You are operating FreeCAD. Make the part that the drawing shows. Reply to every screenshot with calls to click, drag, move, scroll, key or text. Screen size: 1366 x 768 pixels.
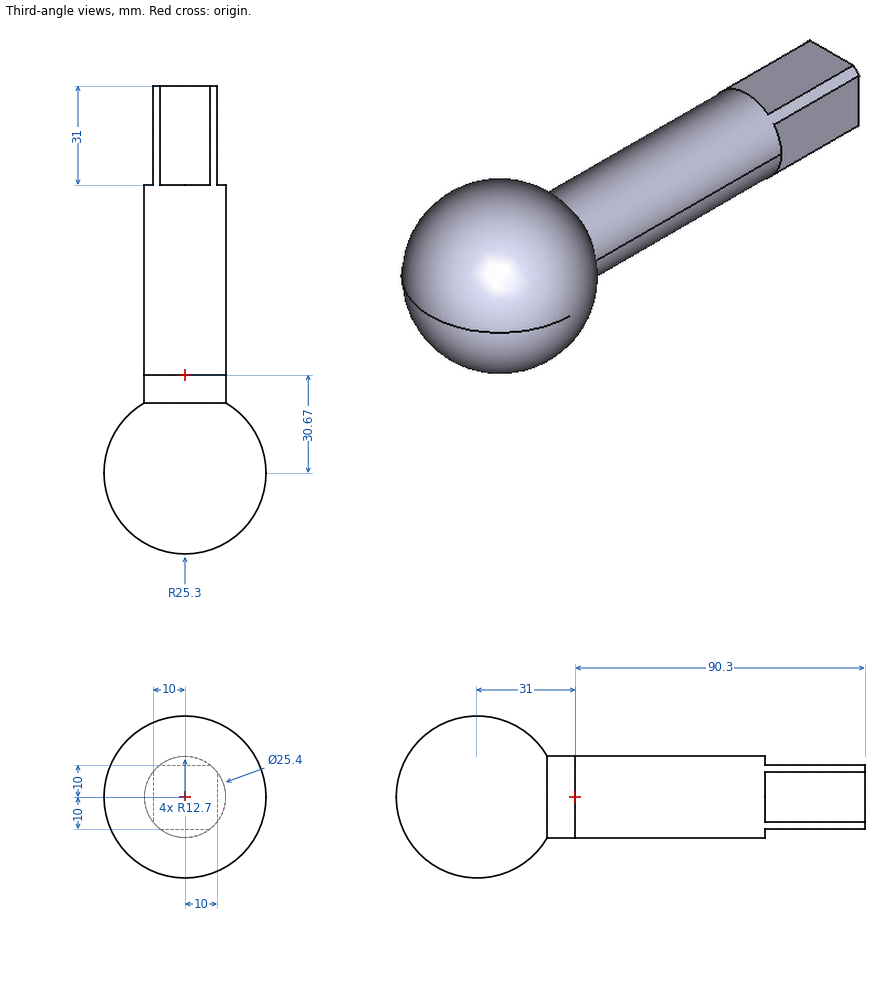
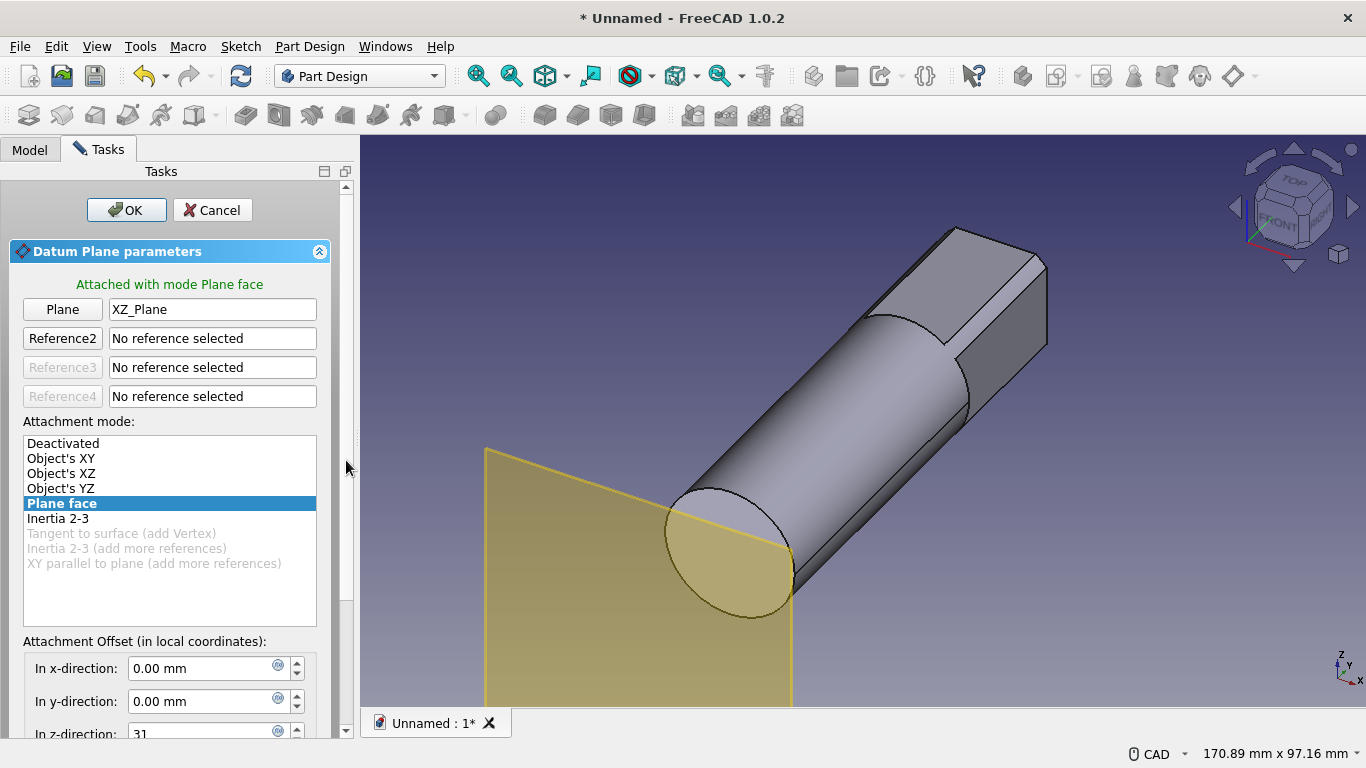
click(127, 210)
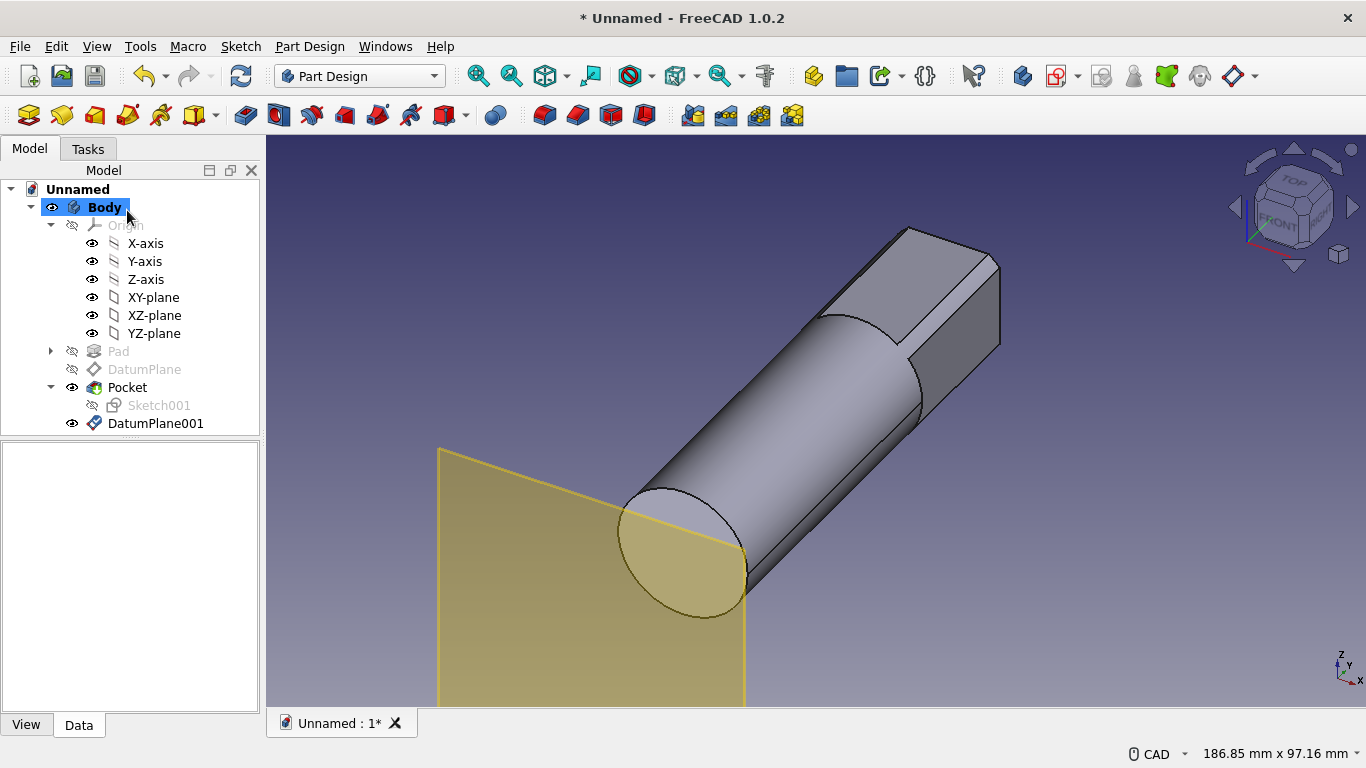
click(117, 423)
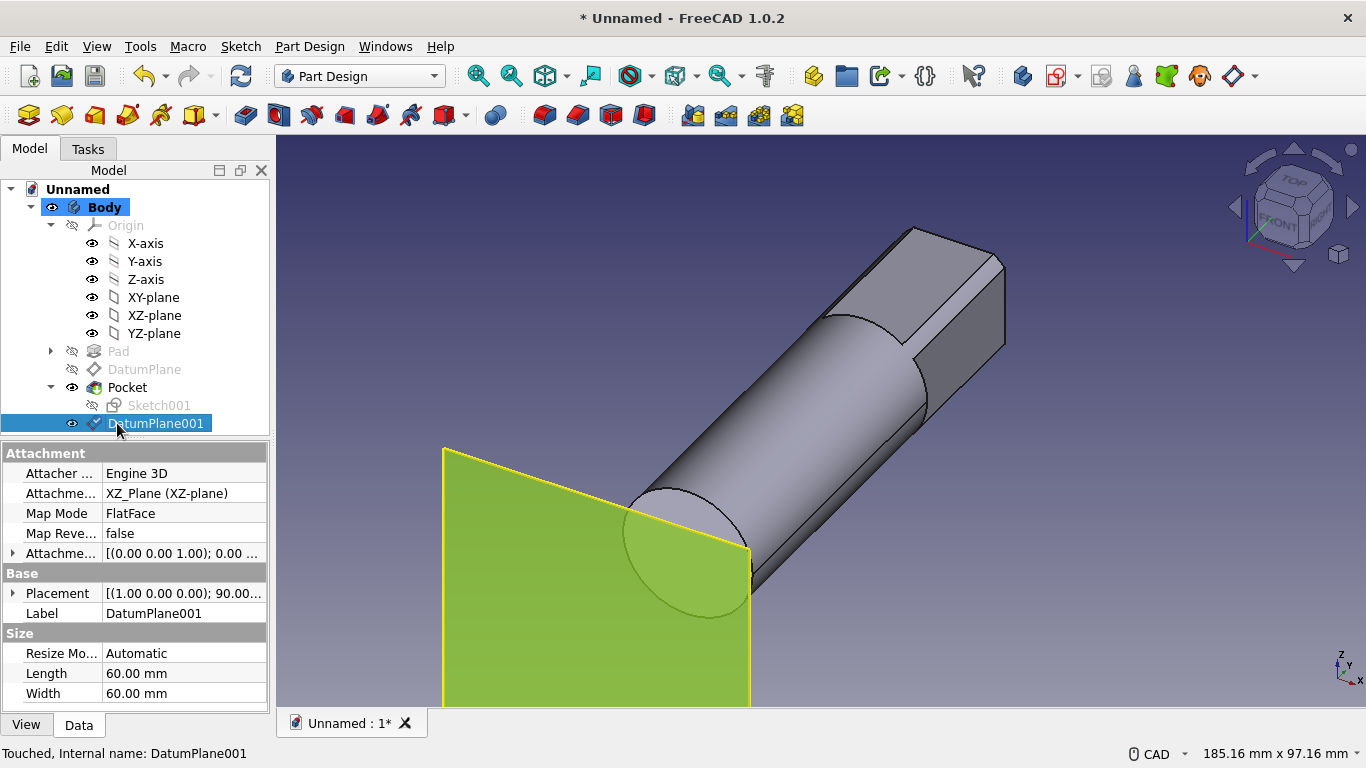
click(1056, 76)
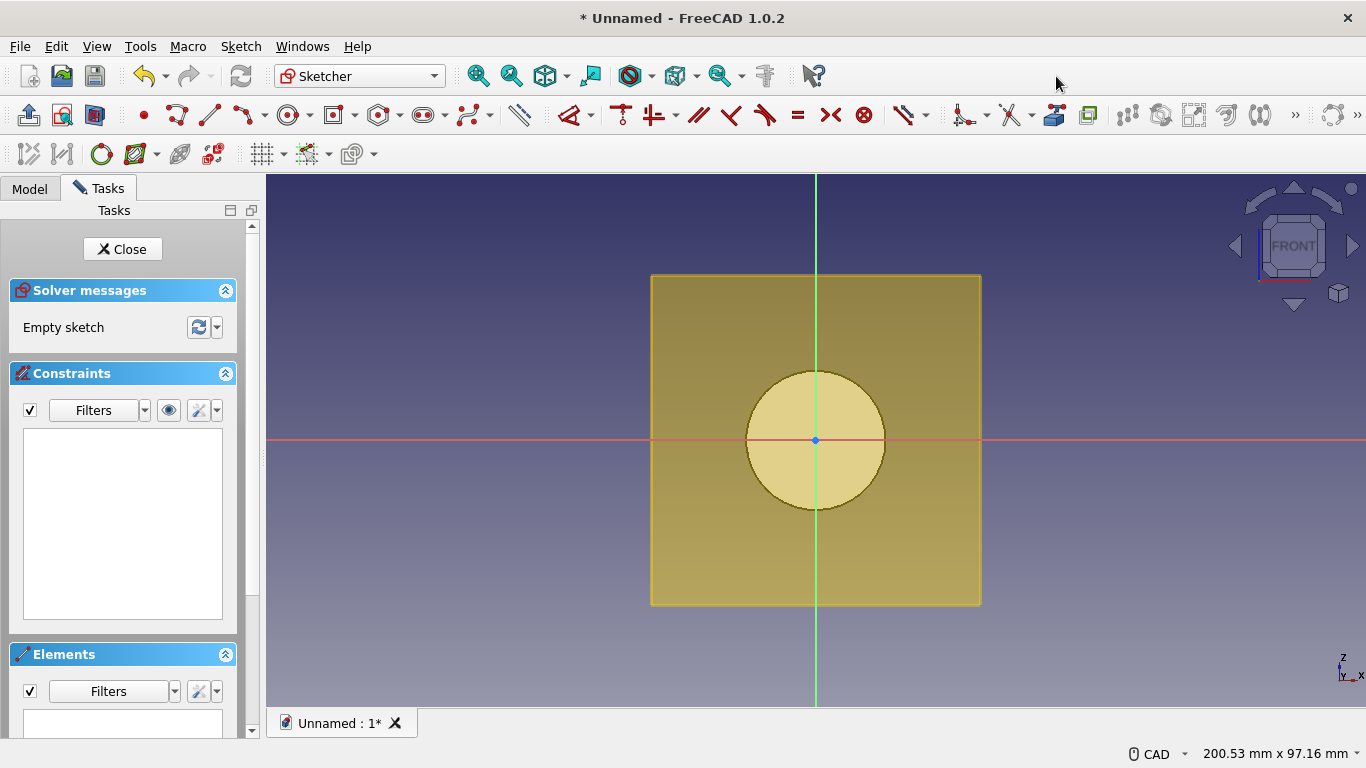
scroll(872, 440, up, 4)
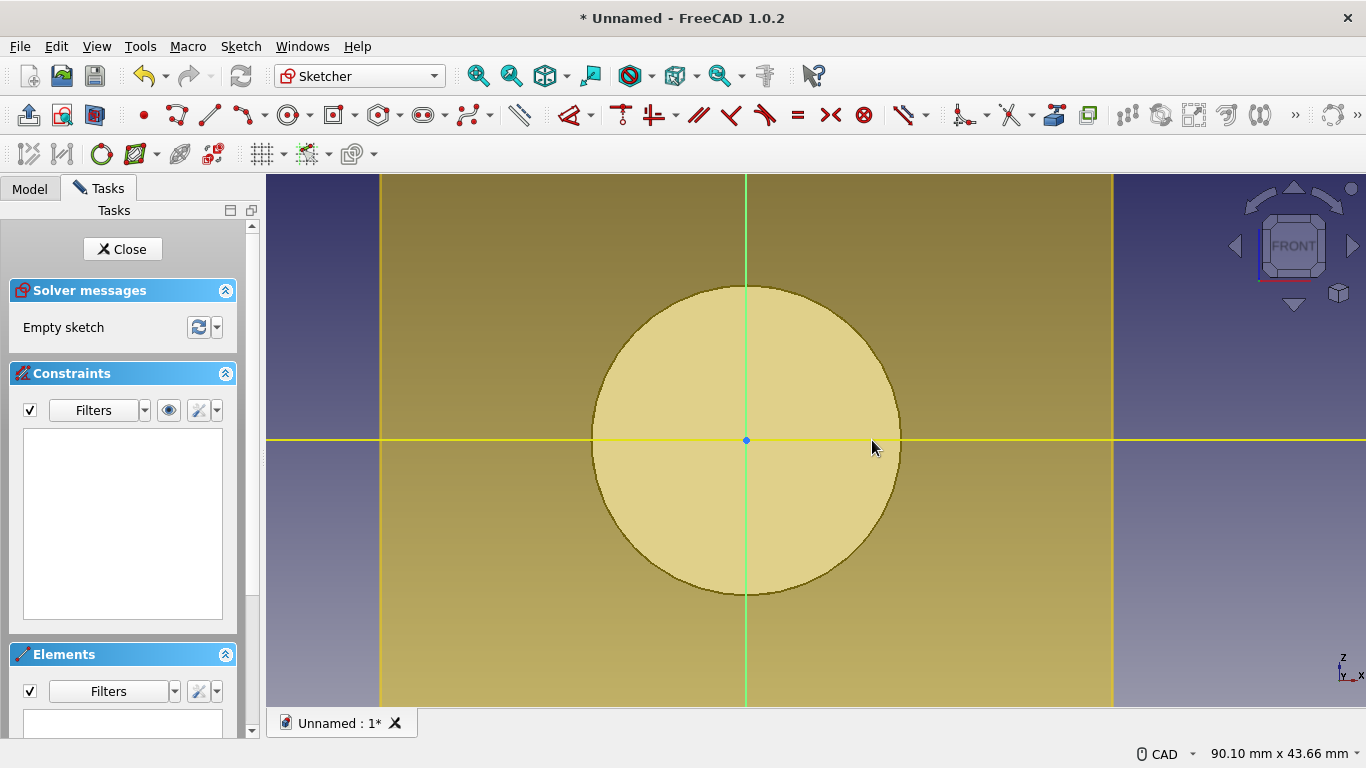
click(288, 116)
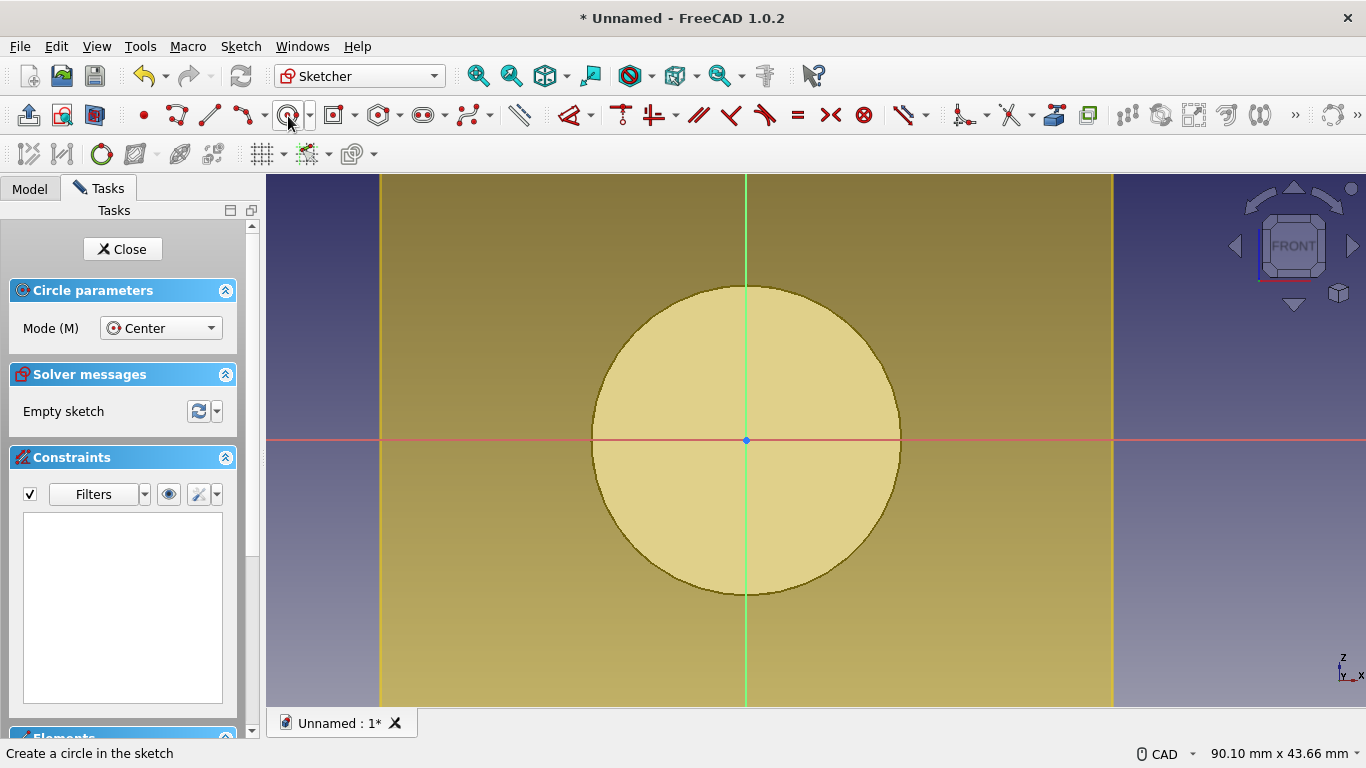
click(746, 440)
move(856, 331)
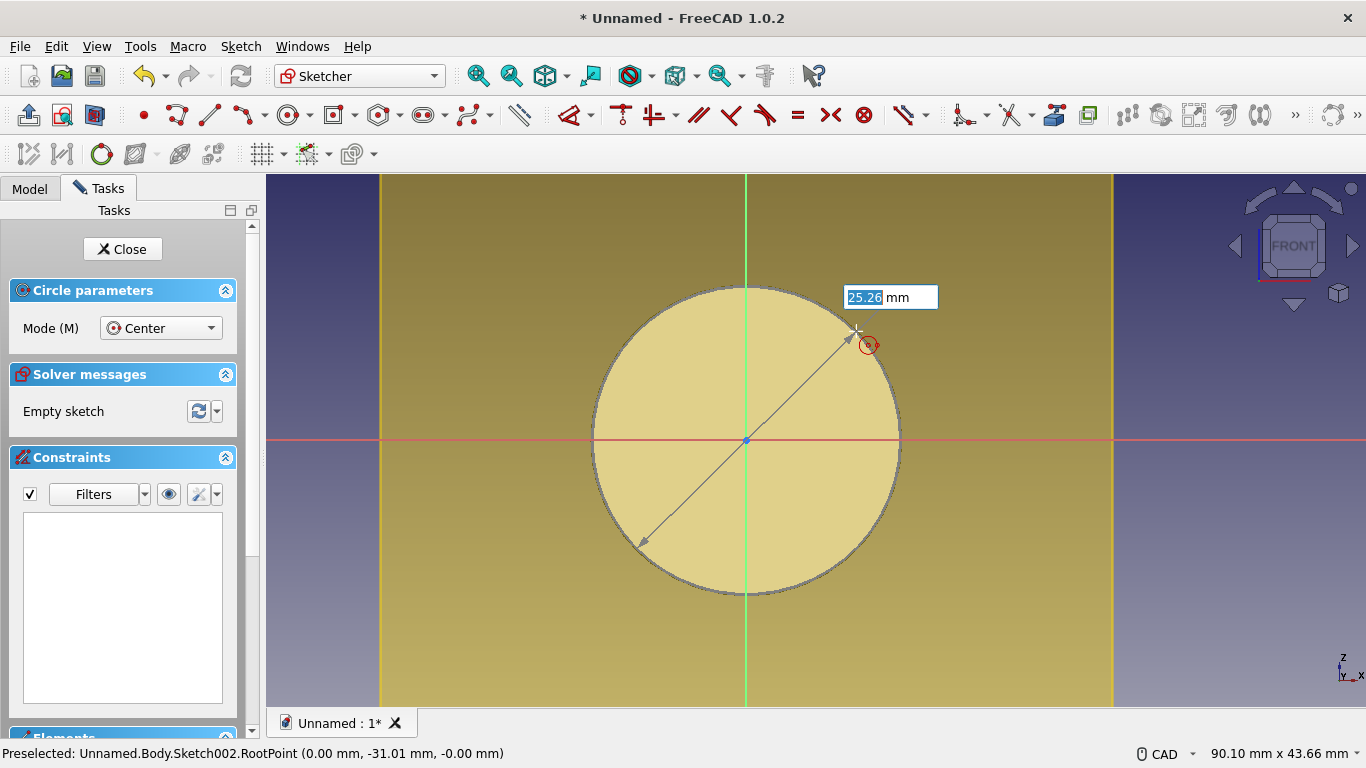
text(25.4)
key(Return)
key(Escape)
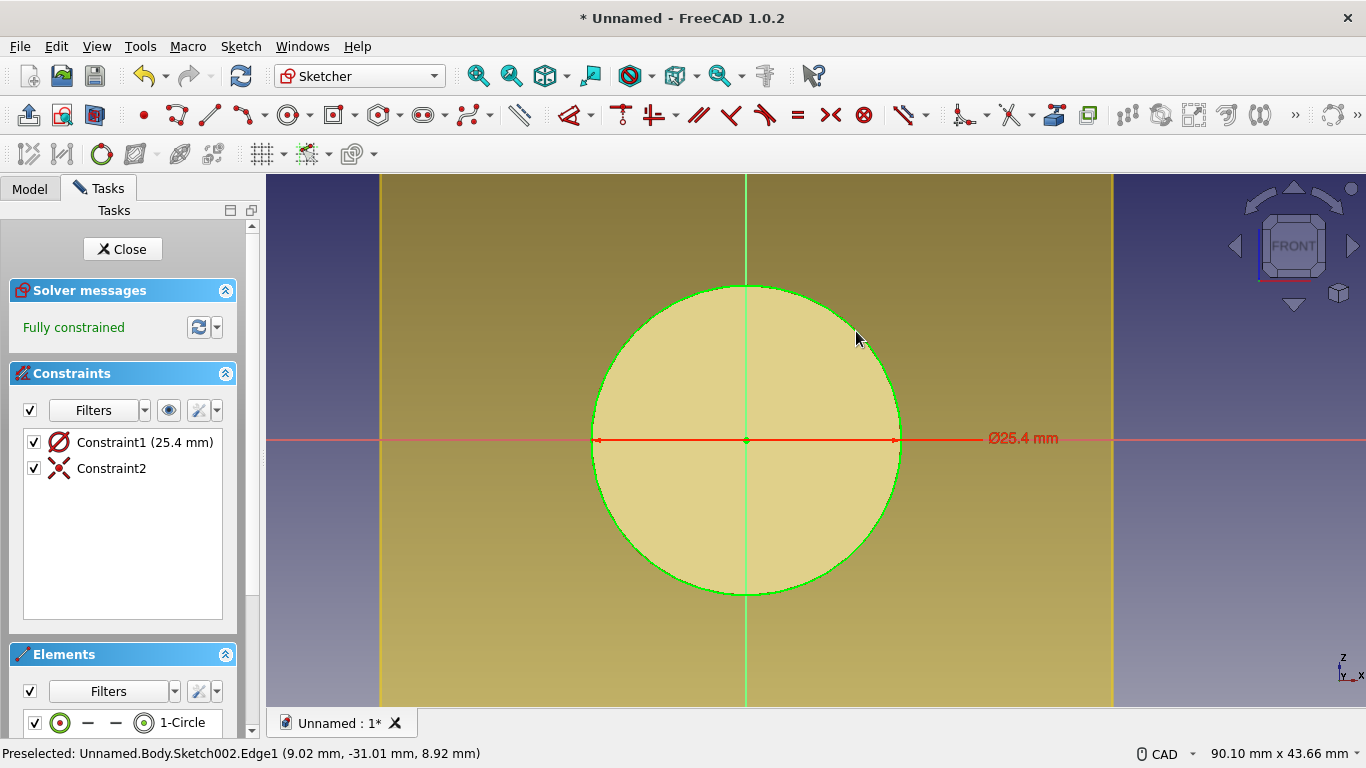
click(123, 249)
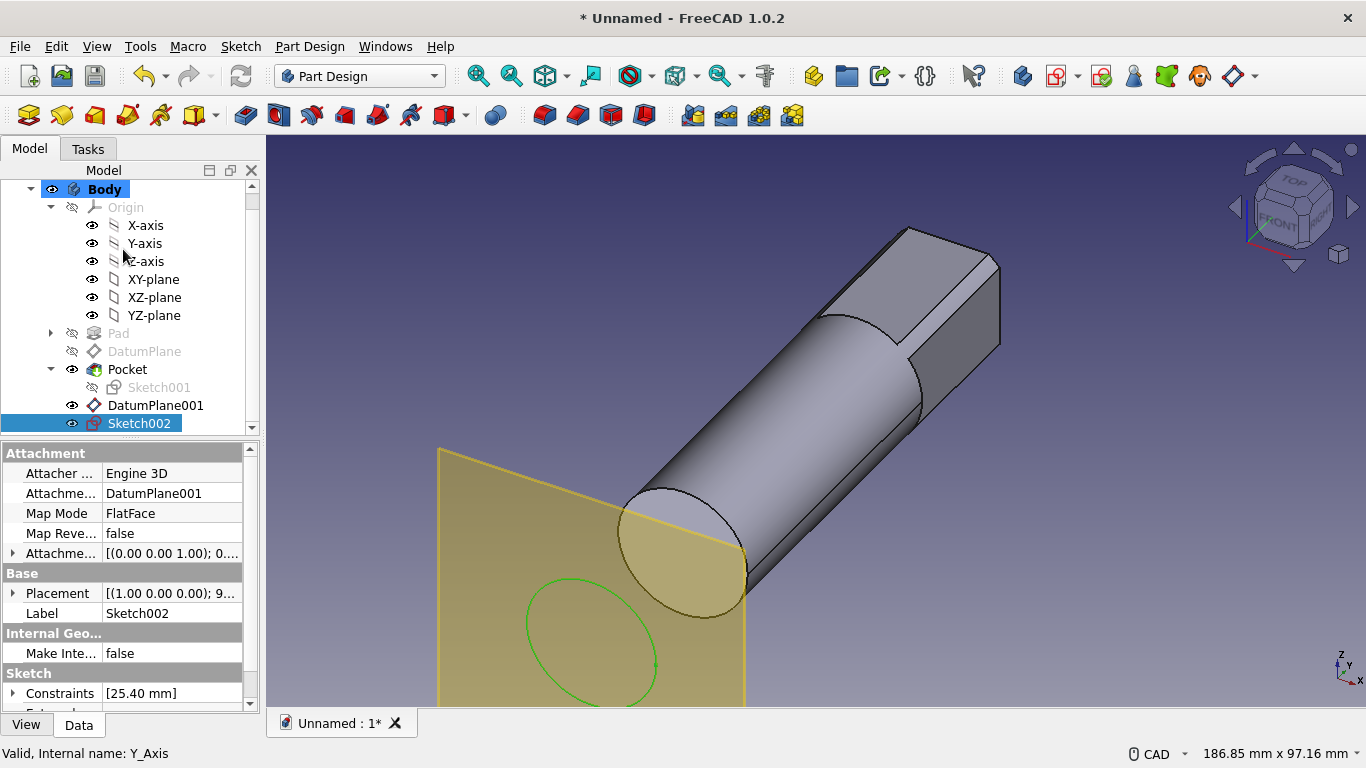
click(29, 116)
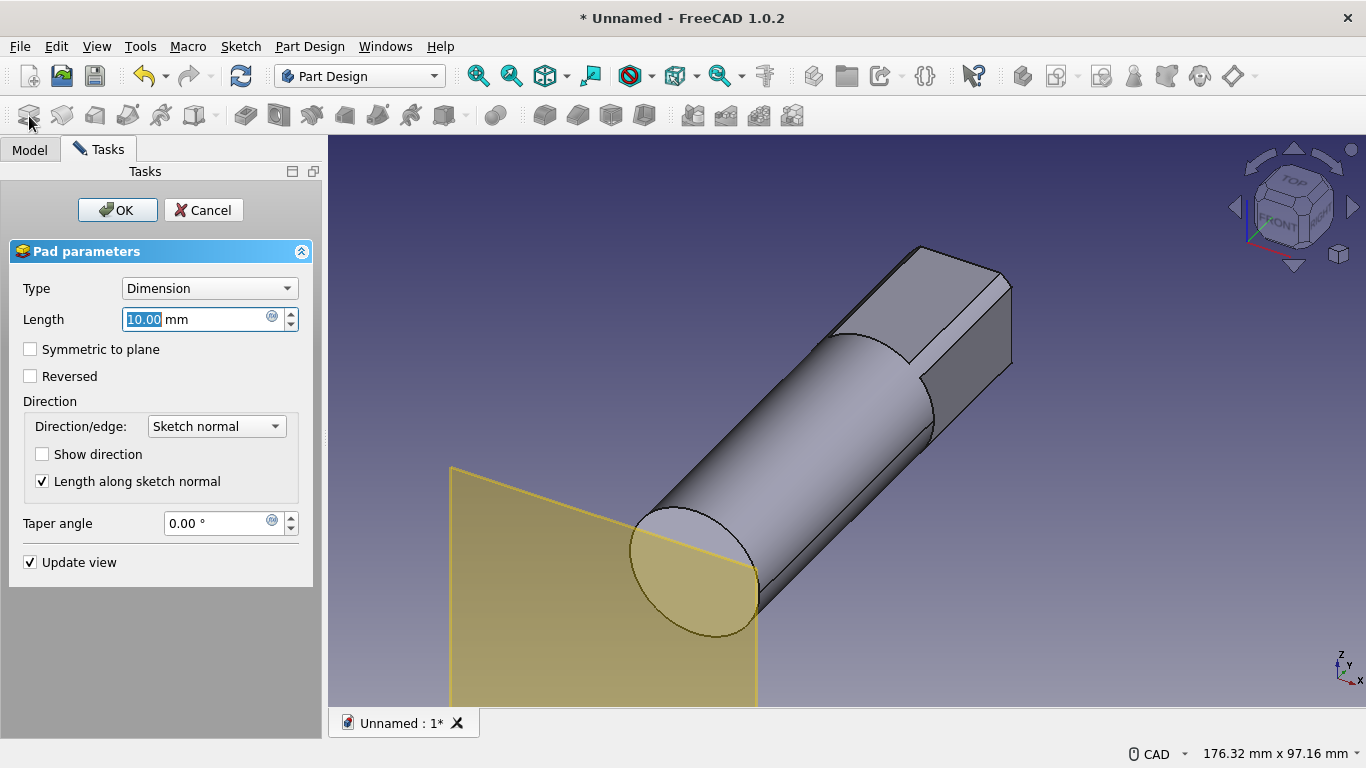
text(31)
key(Tab)